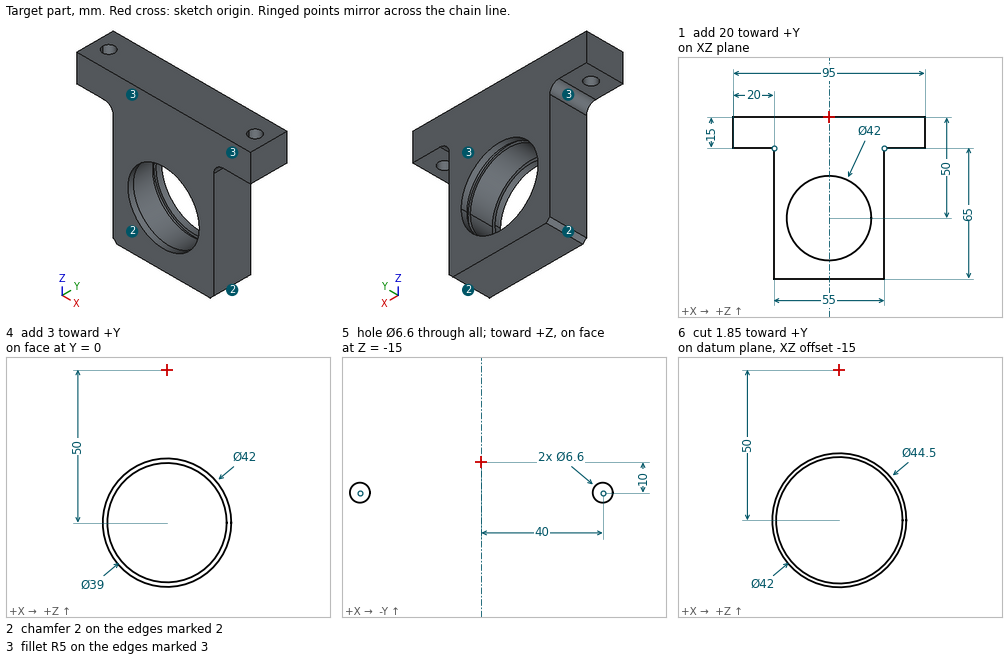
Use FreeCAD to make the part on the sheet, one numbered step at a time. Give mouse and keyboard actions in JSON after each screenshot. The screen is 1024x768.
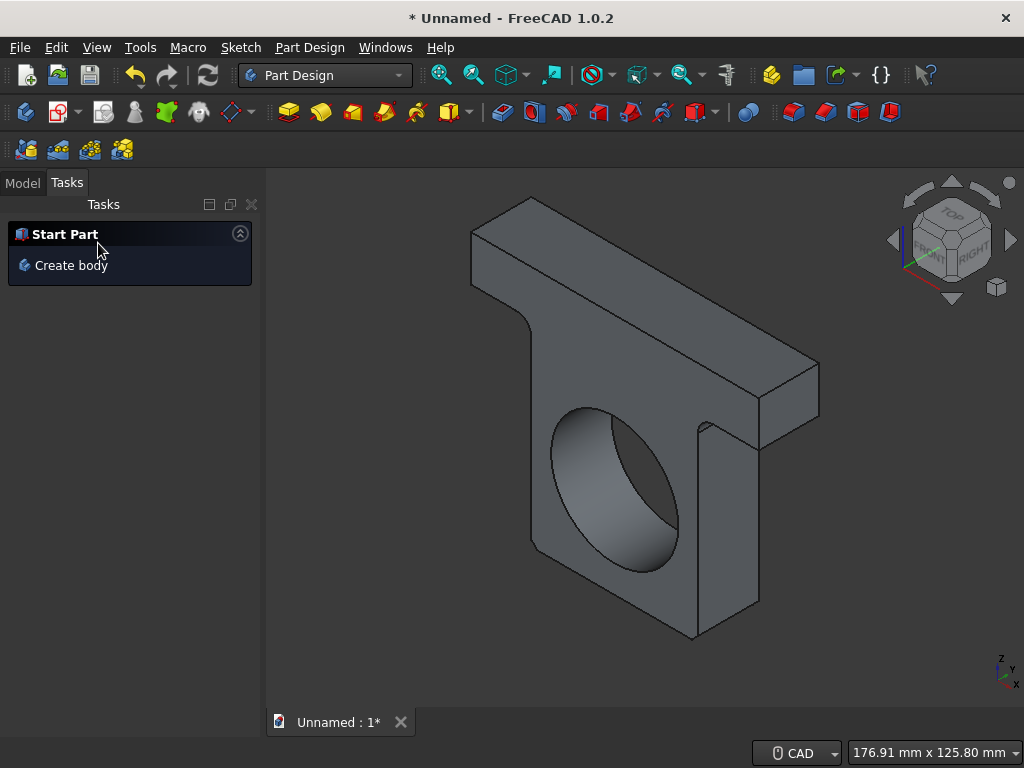
{"action": "left_click", "coordinate": [656, 398]}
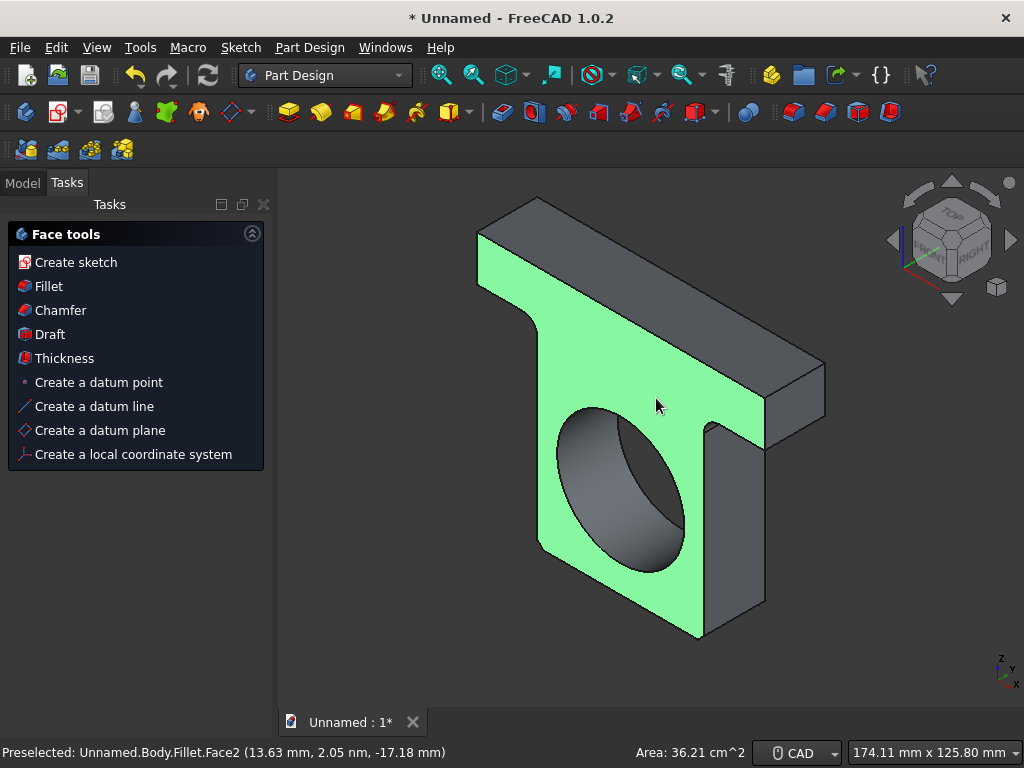
{"action": "left_click", "coordinate": [58, 112]}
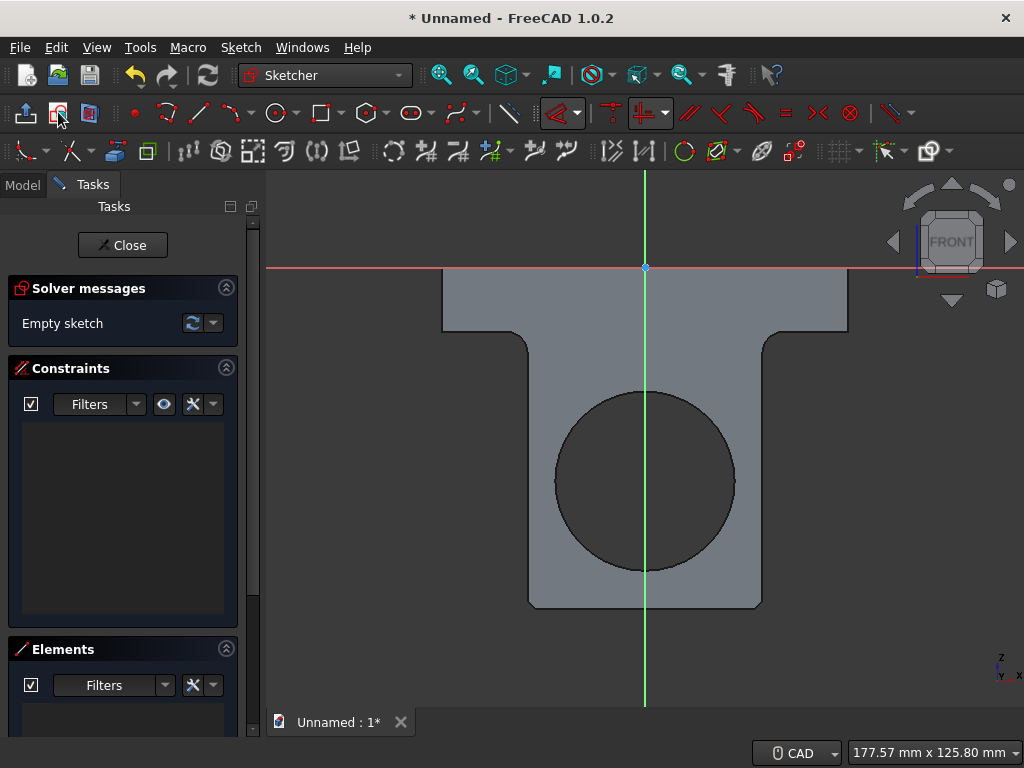
{"action": "left_click", "coordinate": [276, 114]}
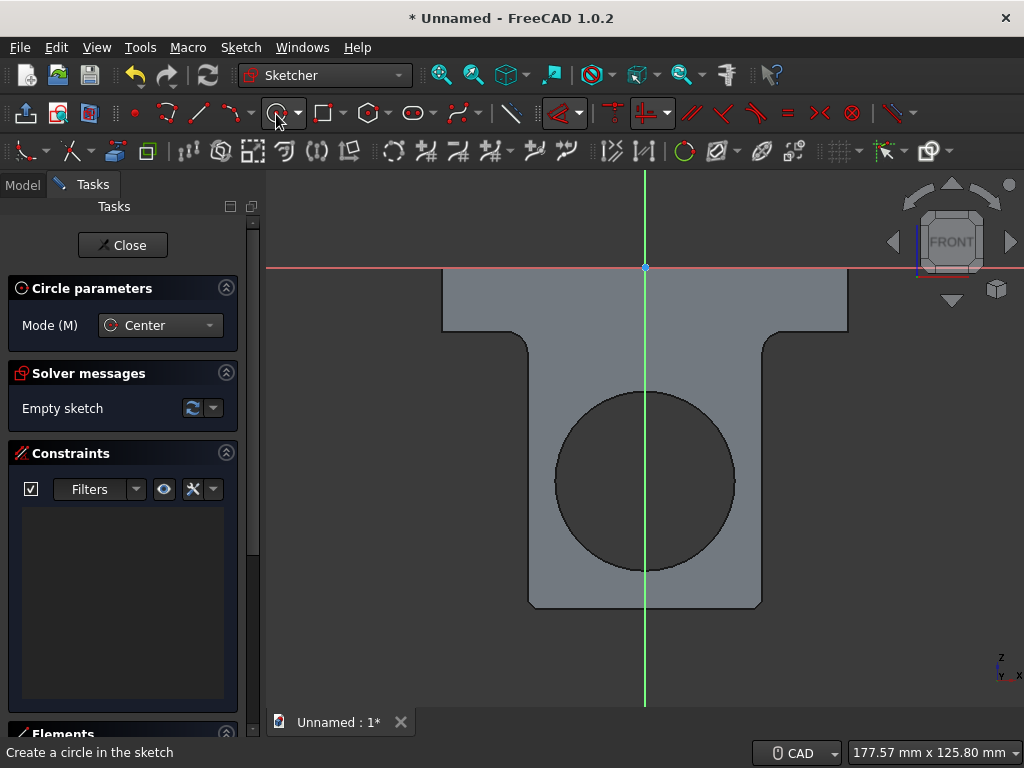
{"action": "left_click", "coordinate": [645, 481]}
{"action": "mouse_move", "coordinate": [708, 418]}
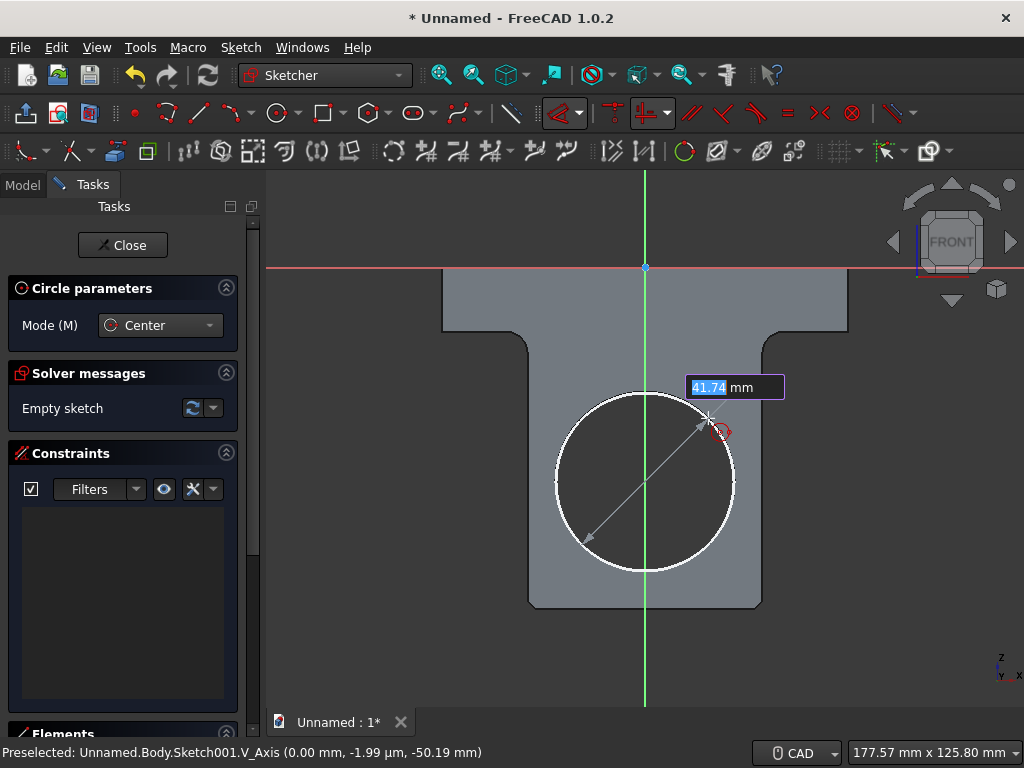
{"action": "type", "text": "42"}
{"action": "key", "text": "Return"}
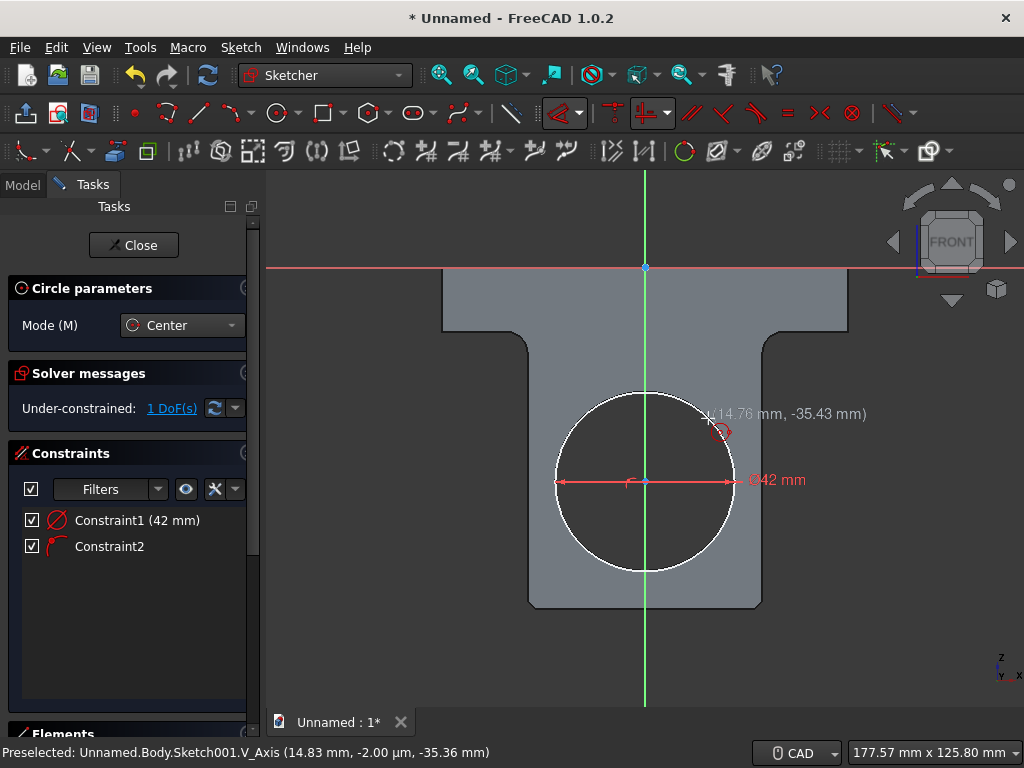
{"action": "left_click", "coordinate": [645, 482]}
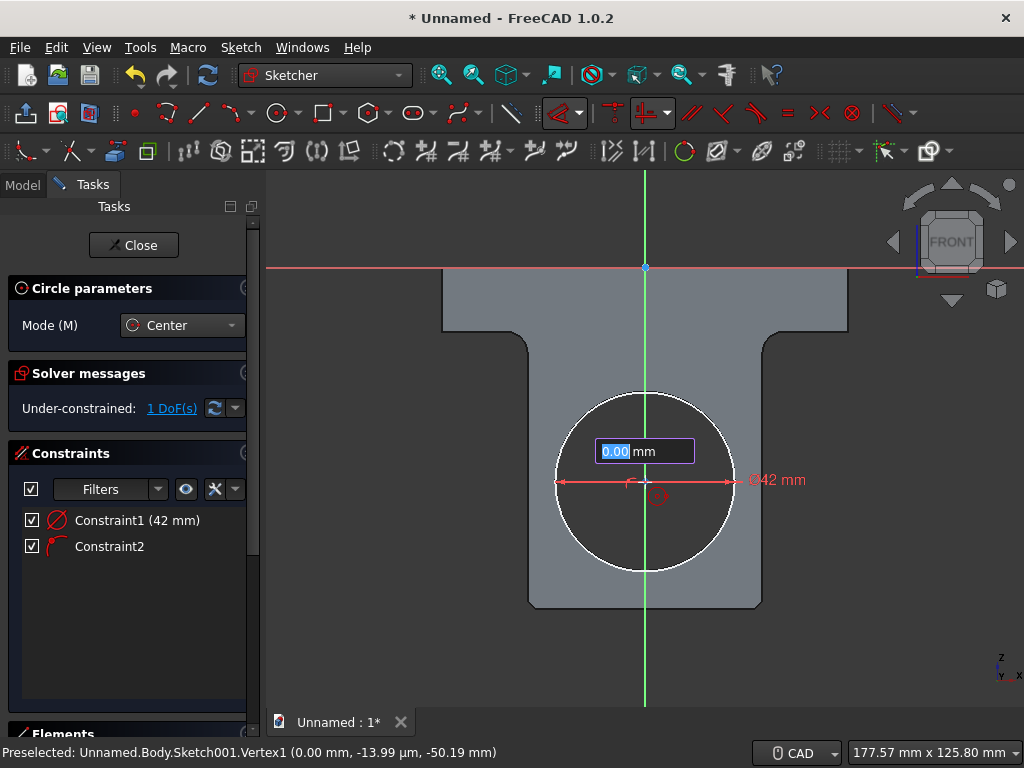
{"action": "scroll", "coordinate": [586, 422], "scroll_direction": "up", "scroll_amount": 5}
{"action": "mouse_move", "coordinate": [586, 422]}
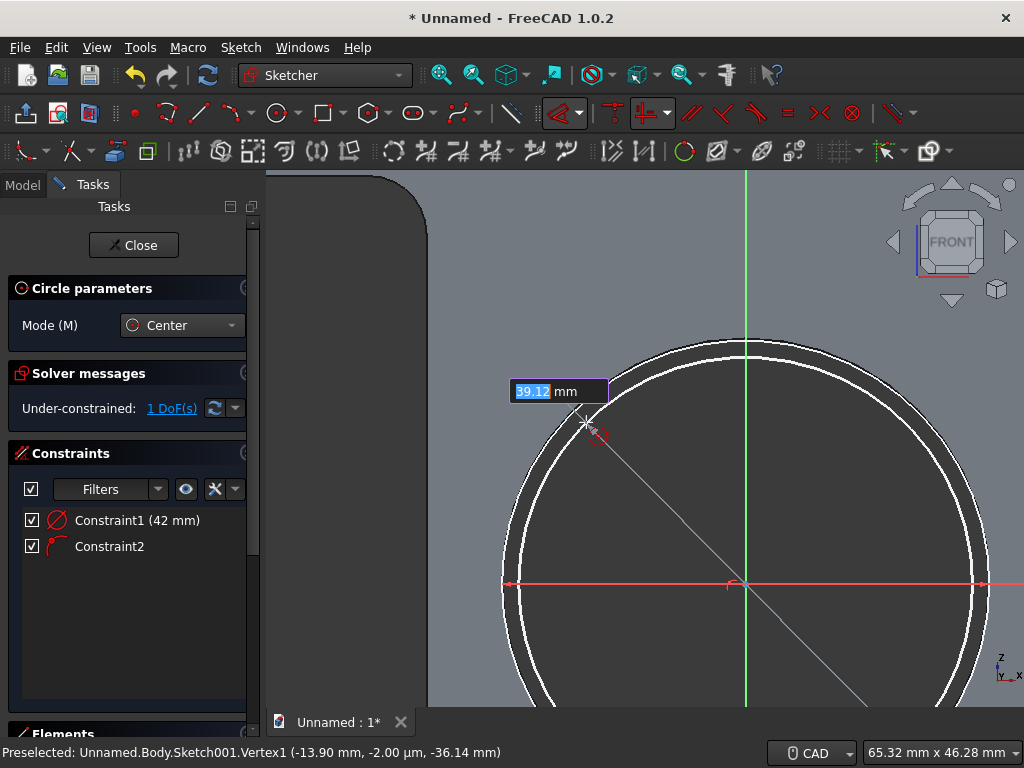
{"action": "type", "text": "39"}
{"action": "key", "text": "Return"}
{"action": "key", "text": "Escape"}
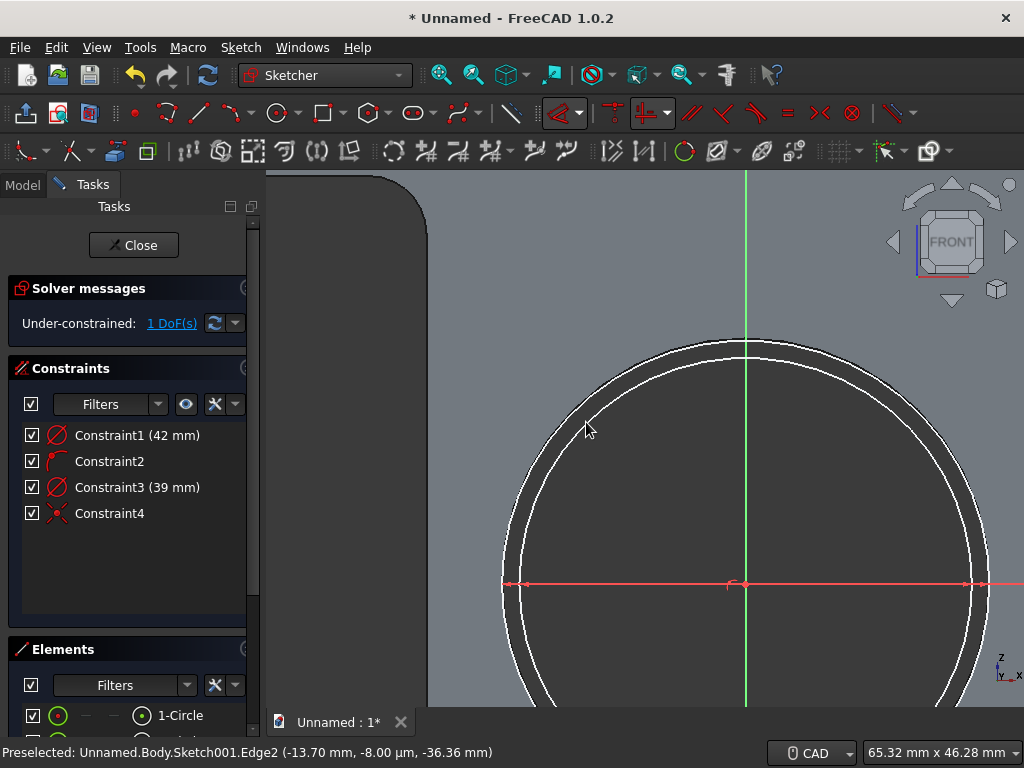
{"action": "left_click", "coordinate": [746, 584]}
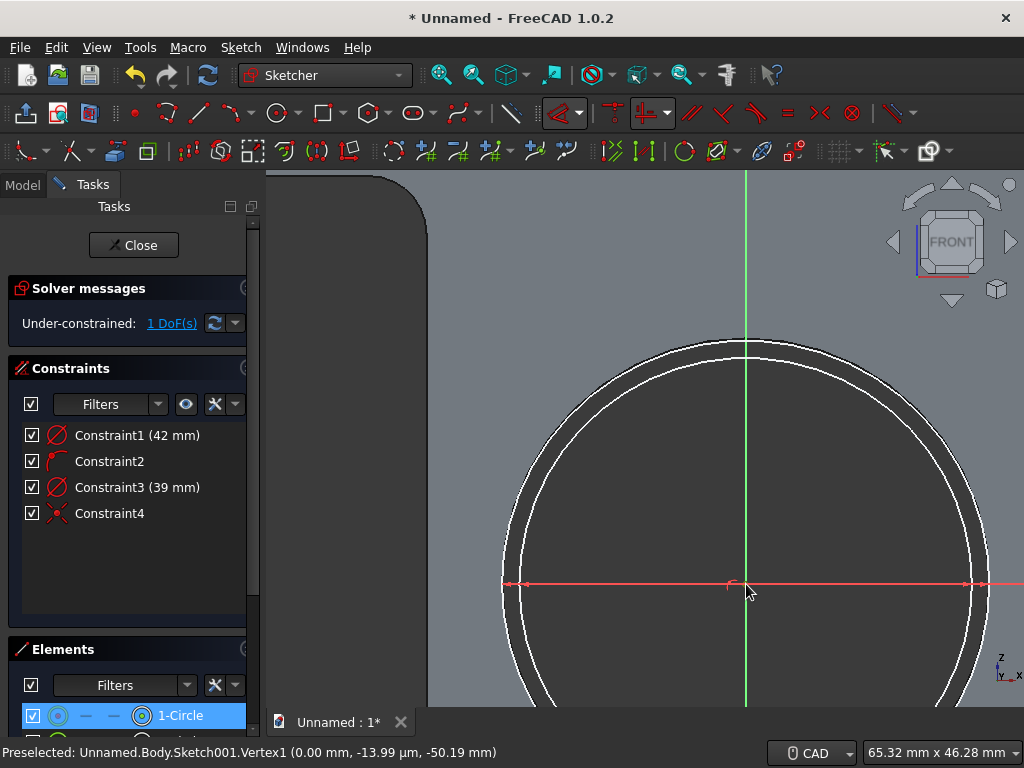
{"action": "left_click", "coordinate": [582, 114]}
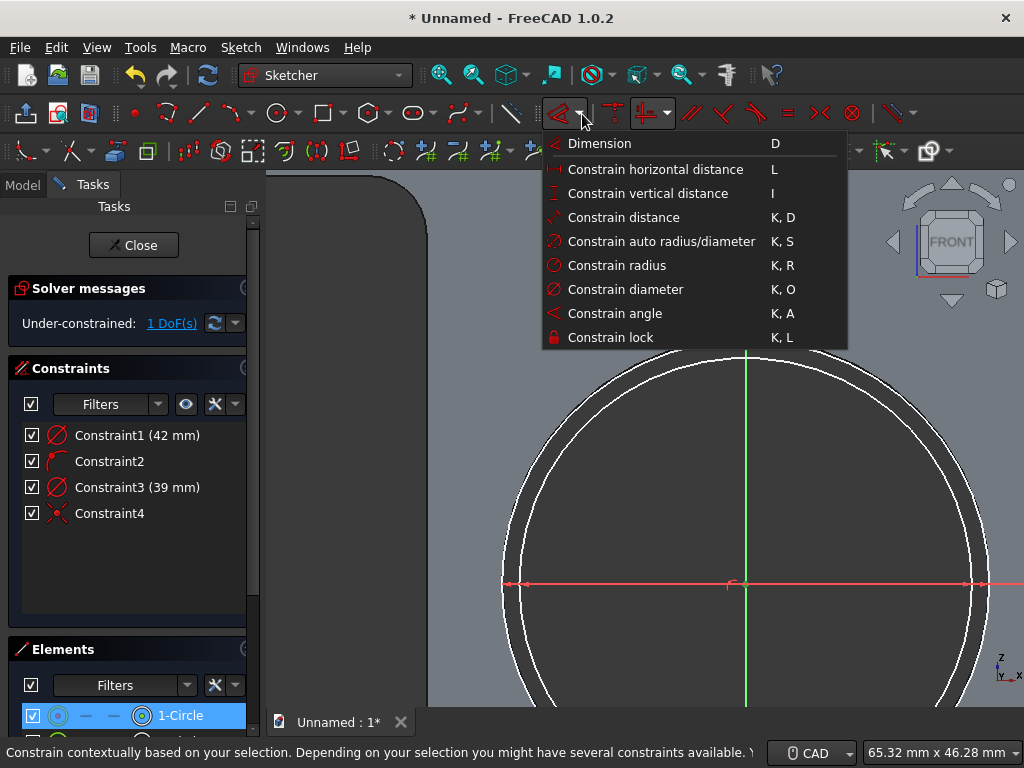
{"action": "left_click", "coordinate": [695, 193]}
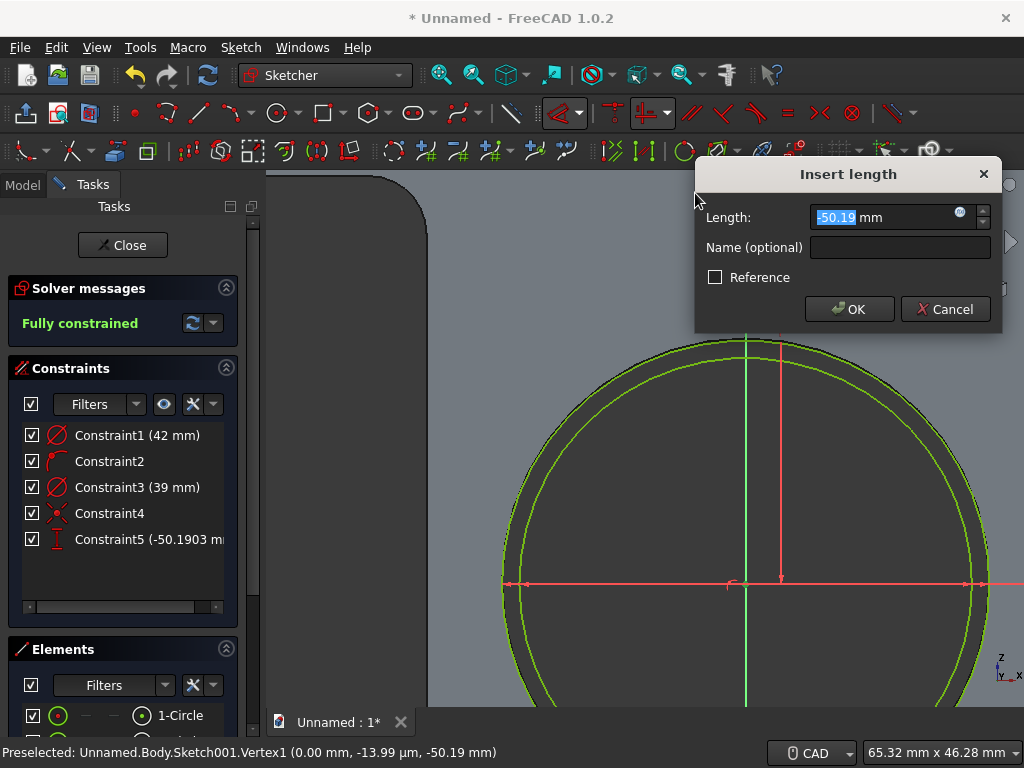
{"action": "type", "text": "-50"}
{"action": "key", "text": "Return"}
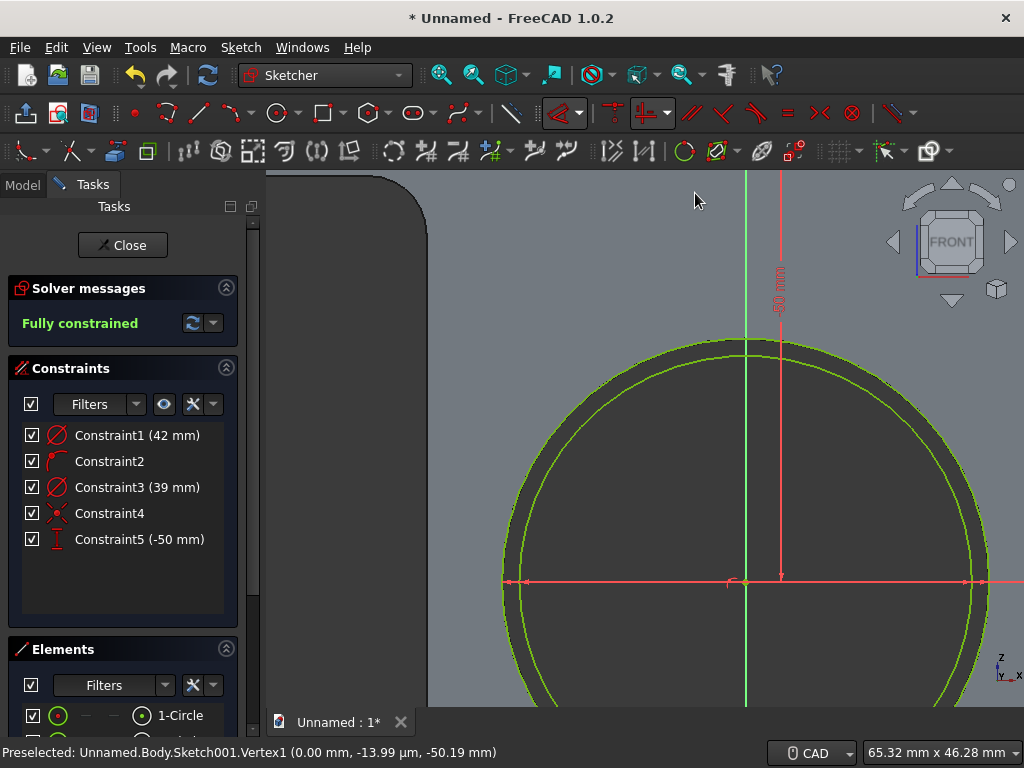
{"action": "left_click", "coordinate": [123, 245]}